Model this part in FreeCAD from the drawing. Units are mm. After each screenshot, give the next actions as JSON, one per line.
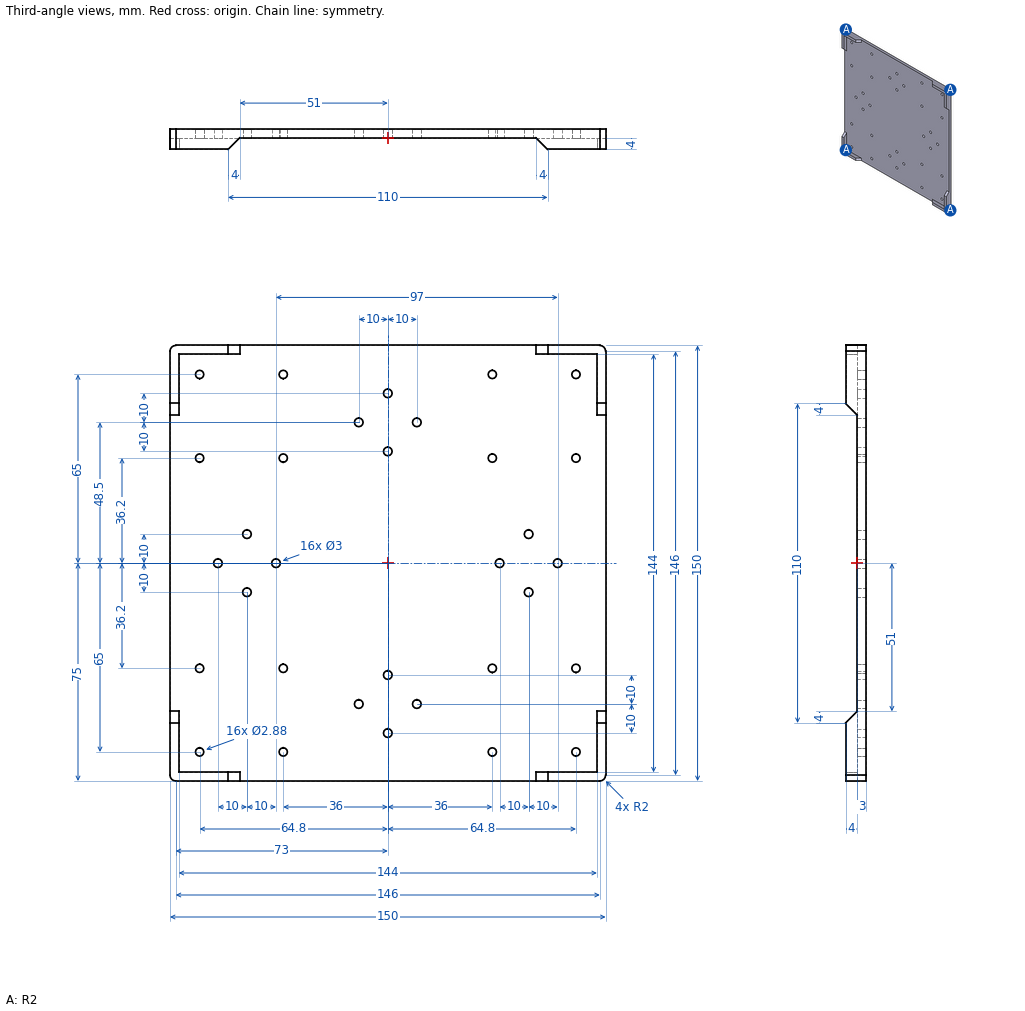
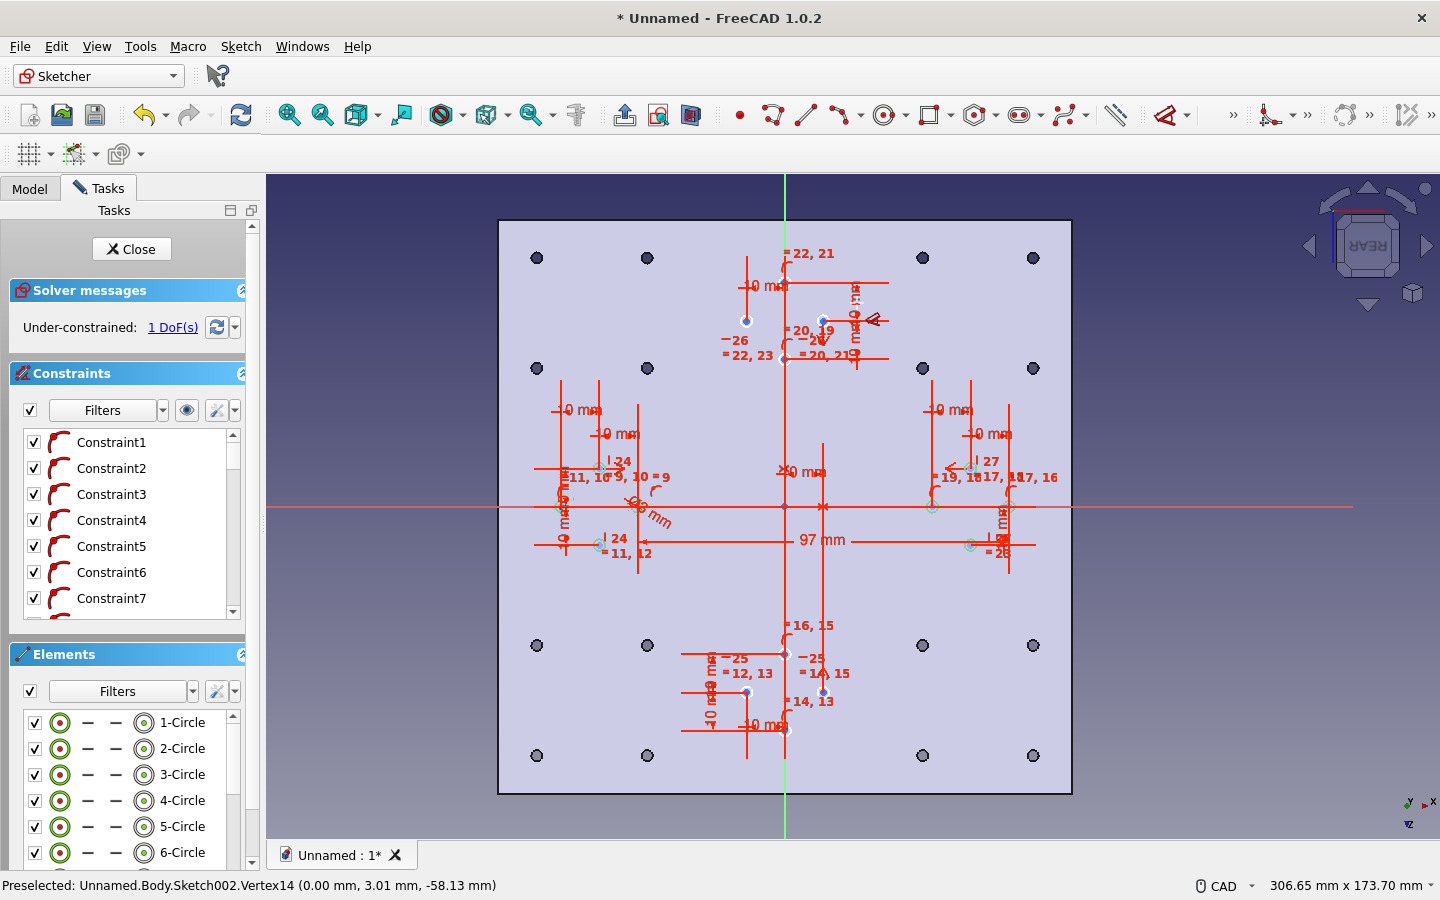
{"action": "left_click", "coordinate": [747, 693]}
{"action": "left_click", "coordinate": [713, 600]}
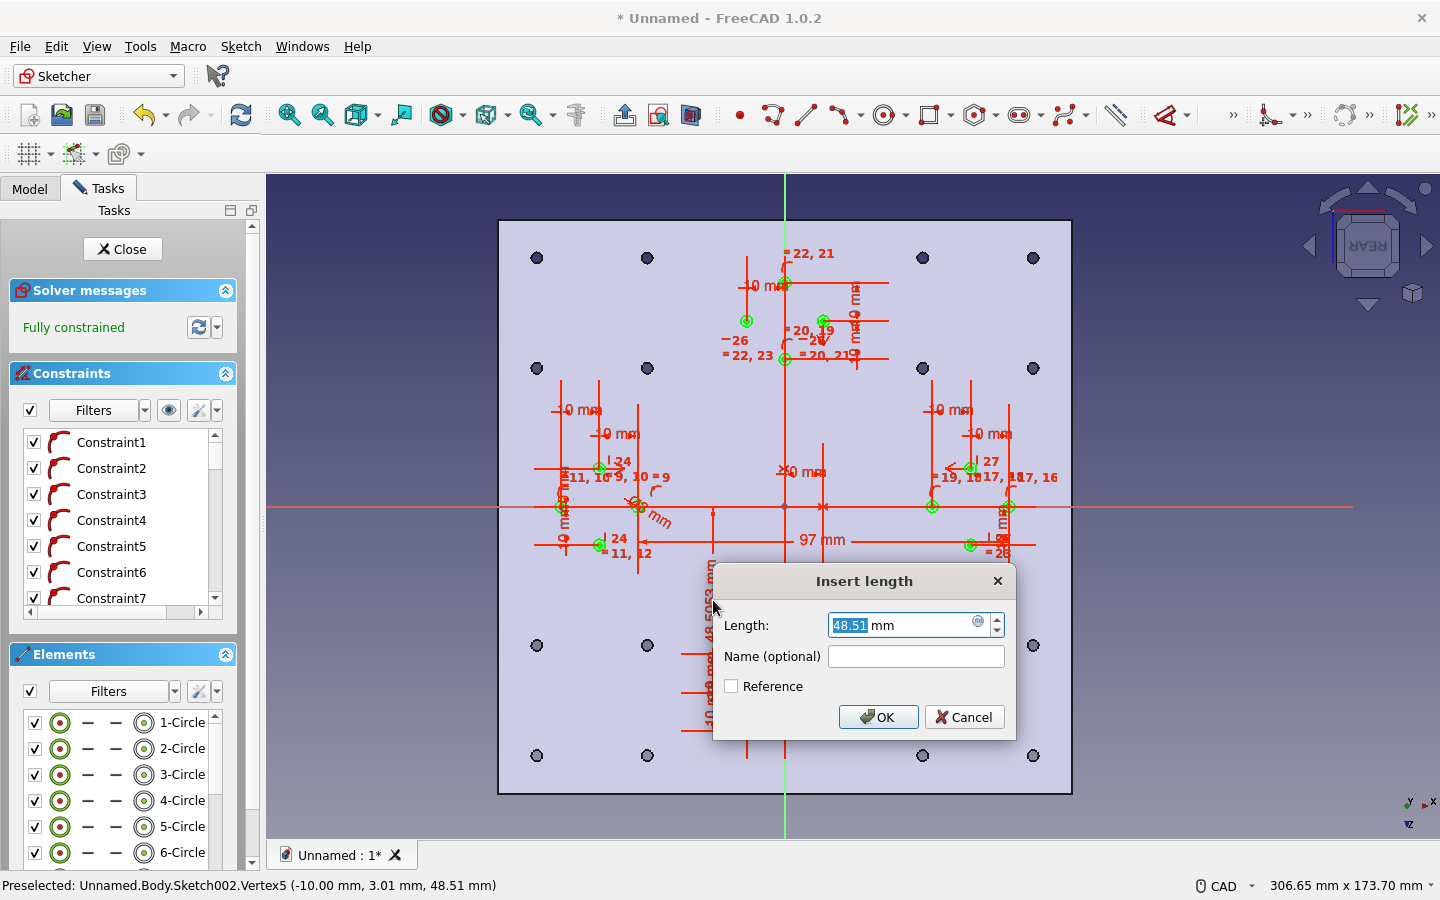
{"action": "type", "text": "48.5"}
{"action": "key", "text": "Return"}
{"action": "key", "text": "Escape"}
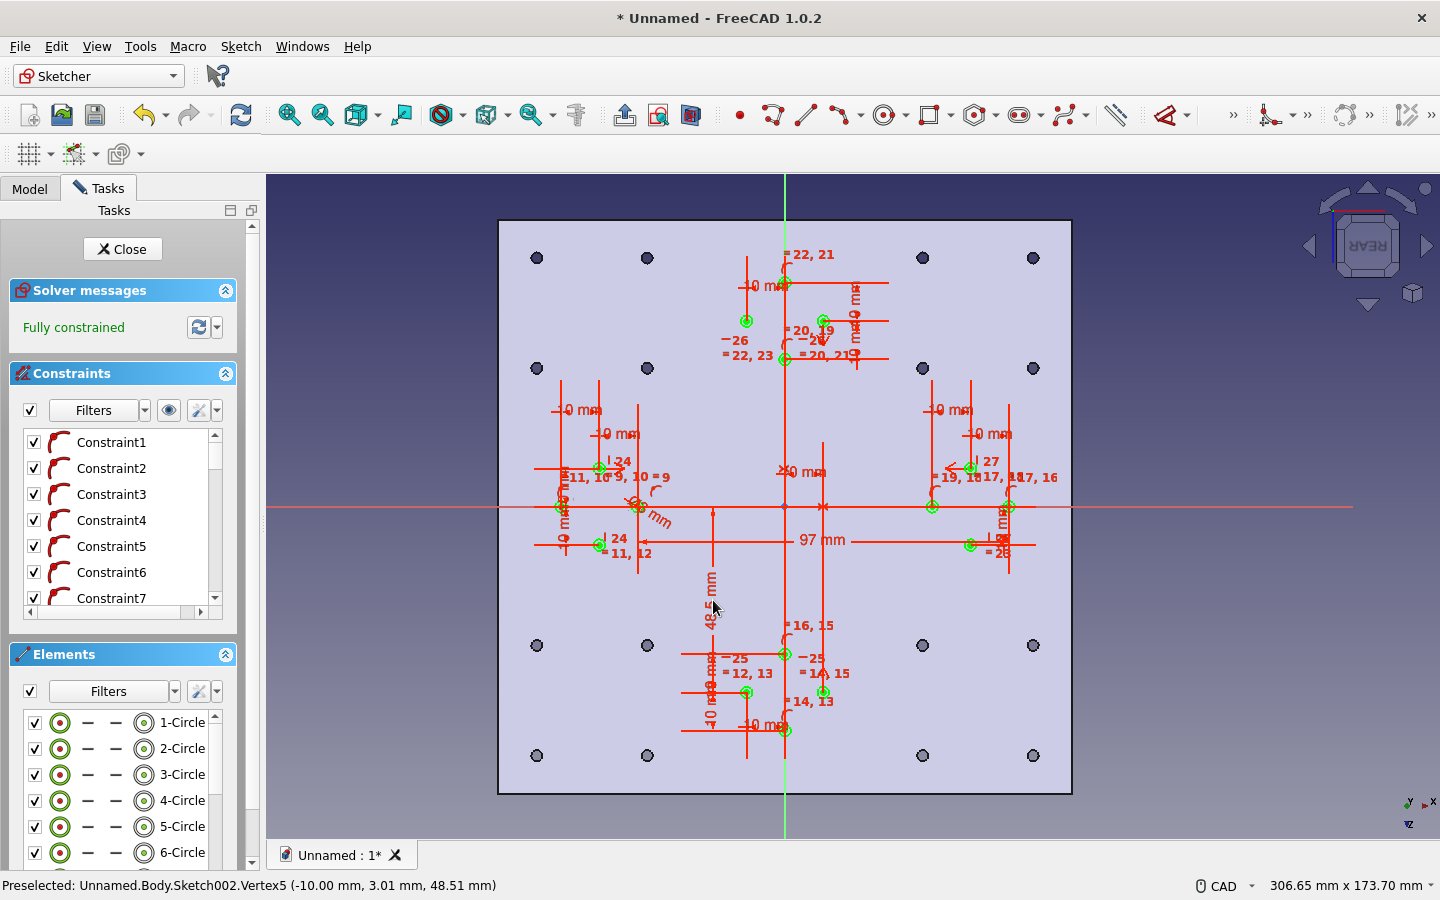
{"action": "left_click", "coordinate": [123, 249]}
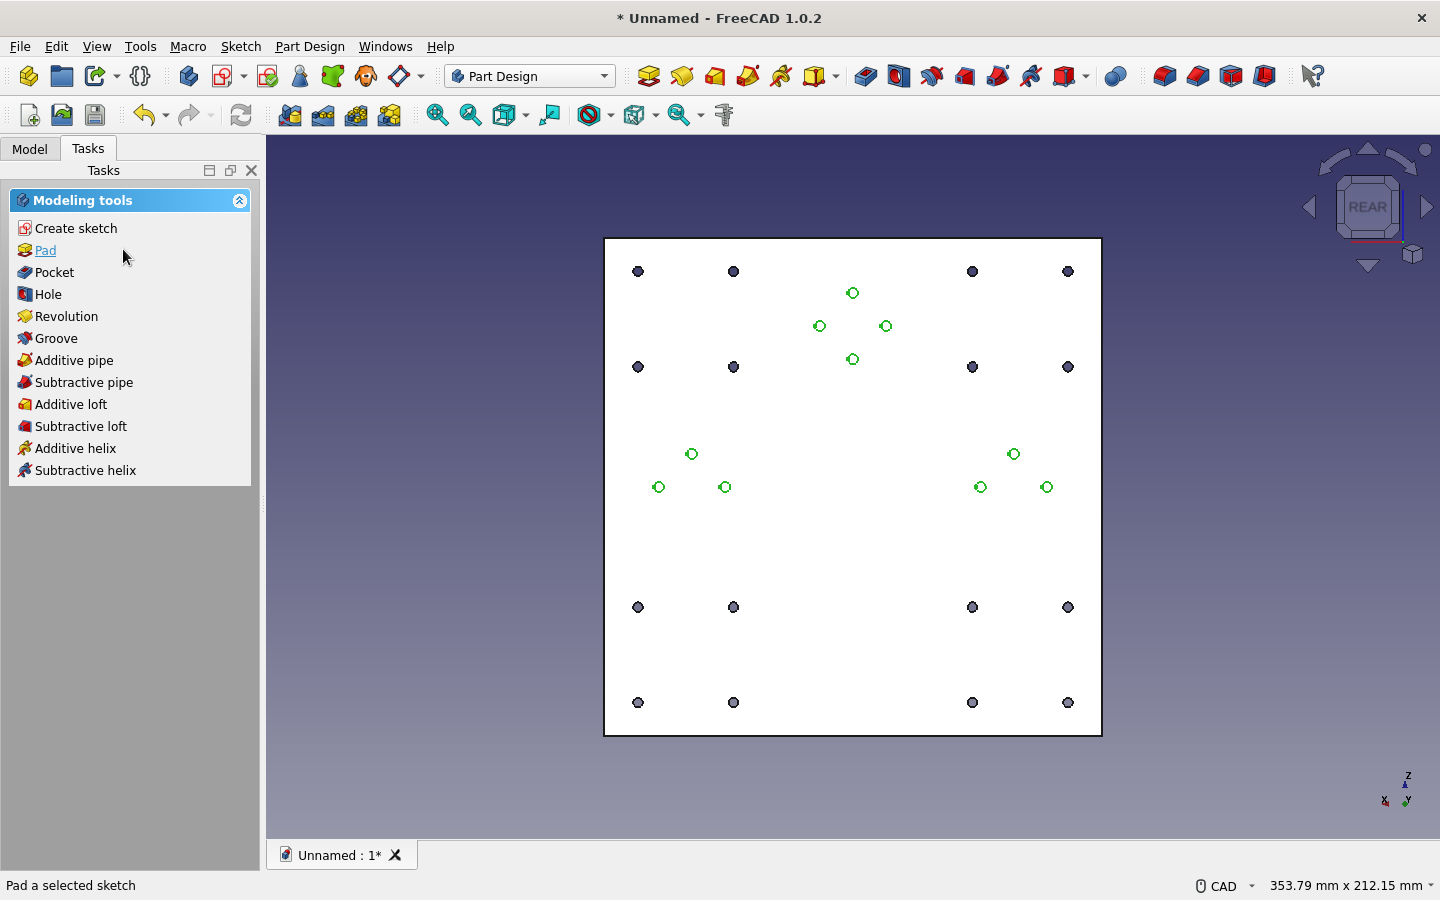
{"action": "left_click", "coordinate": [866, 76]}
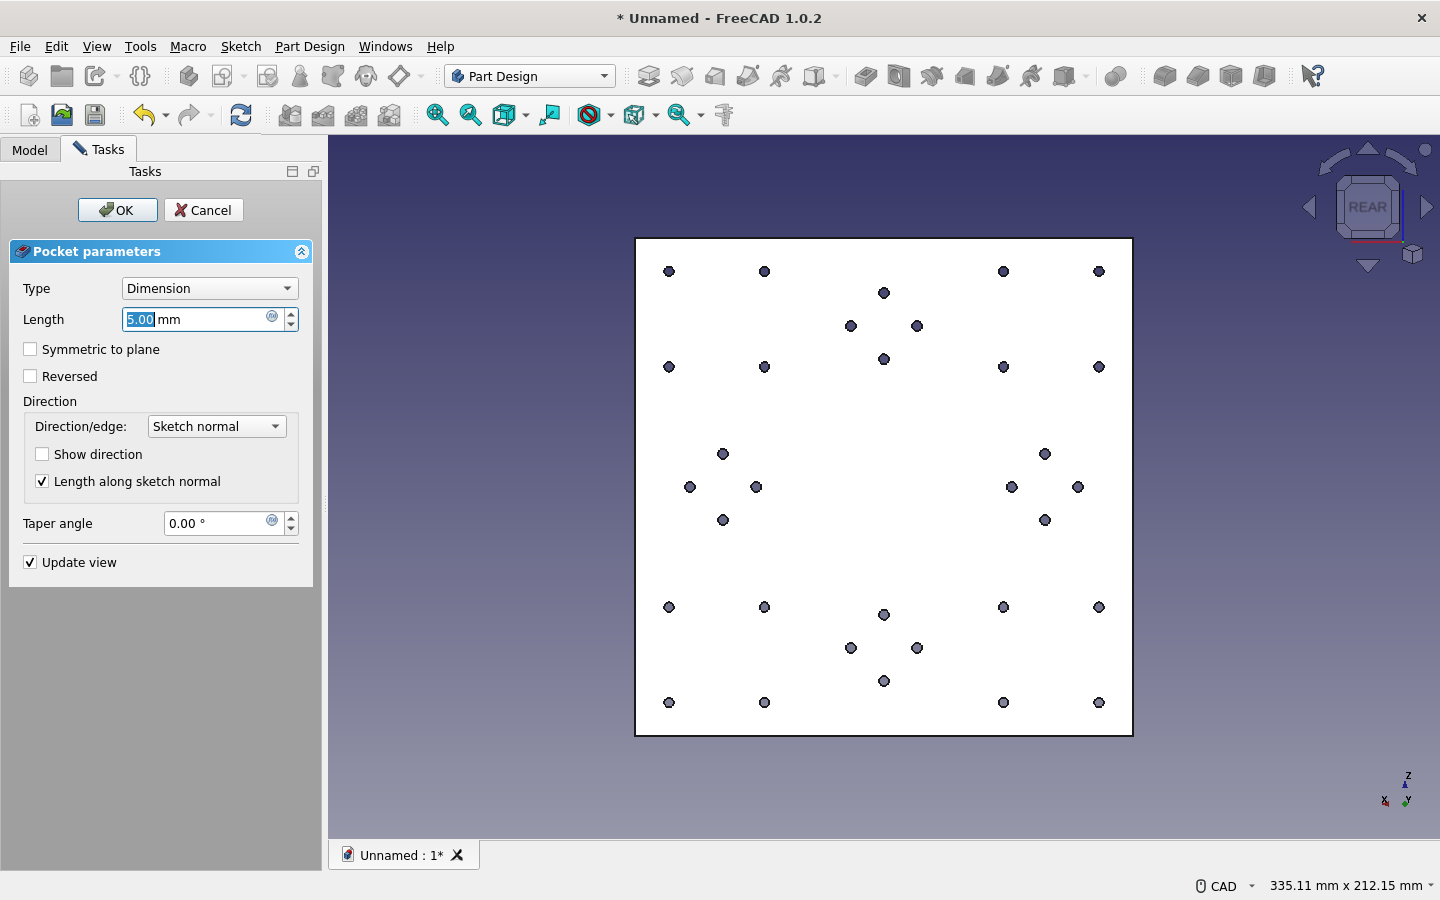
{"action": "left_click", "coordinate": [210, 288]}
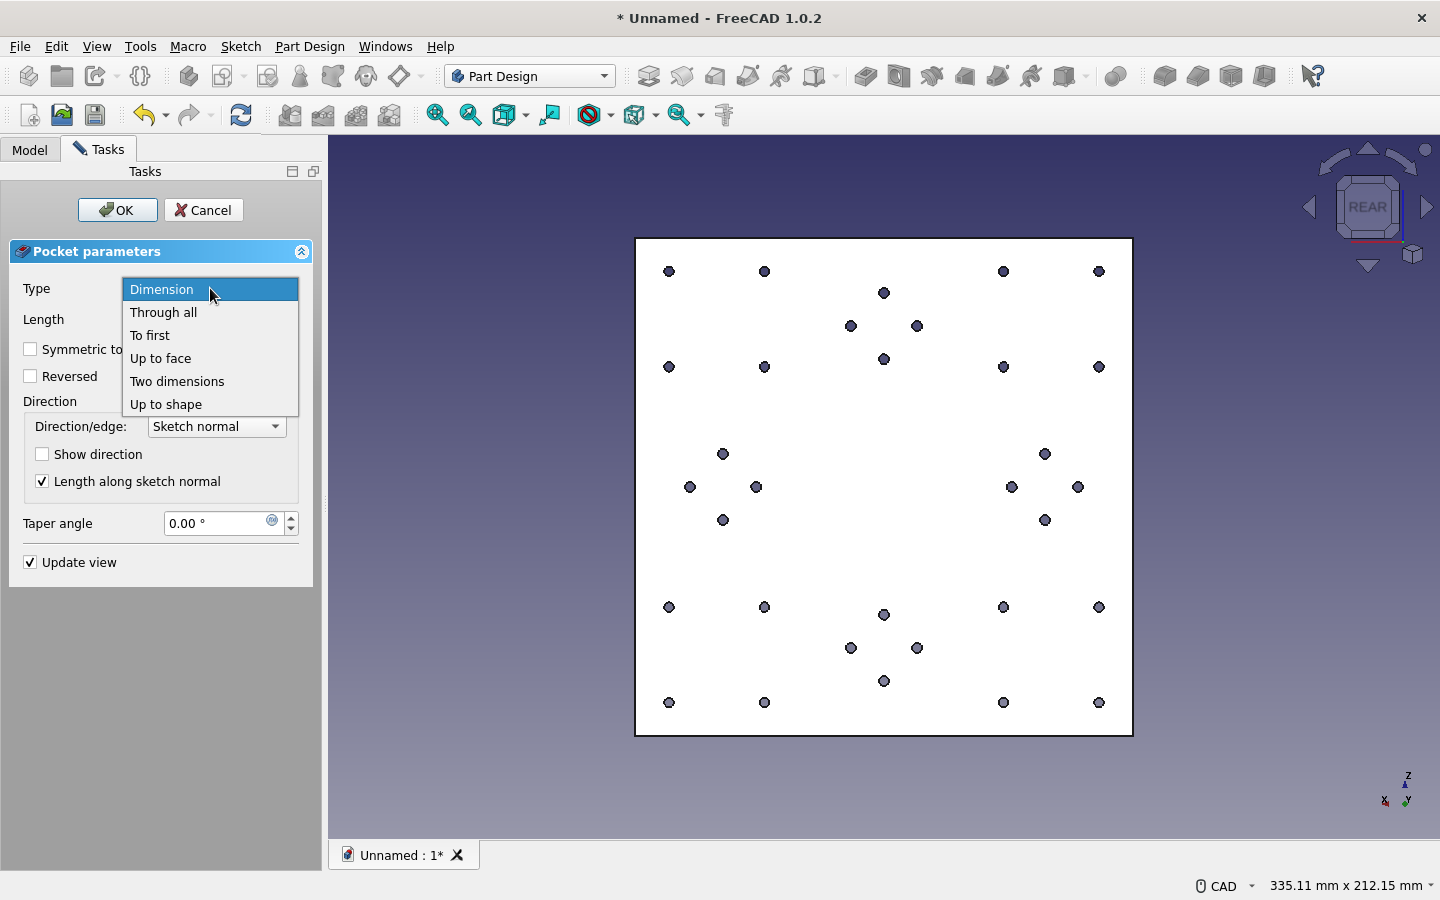
{"action": "left_click", "coordinate": [208, 312]}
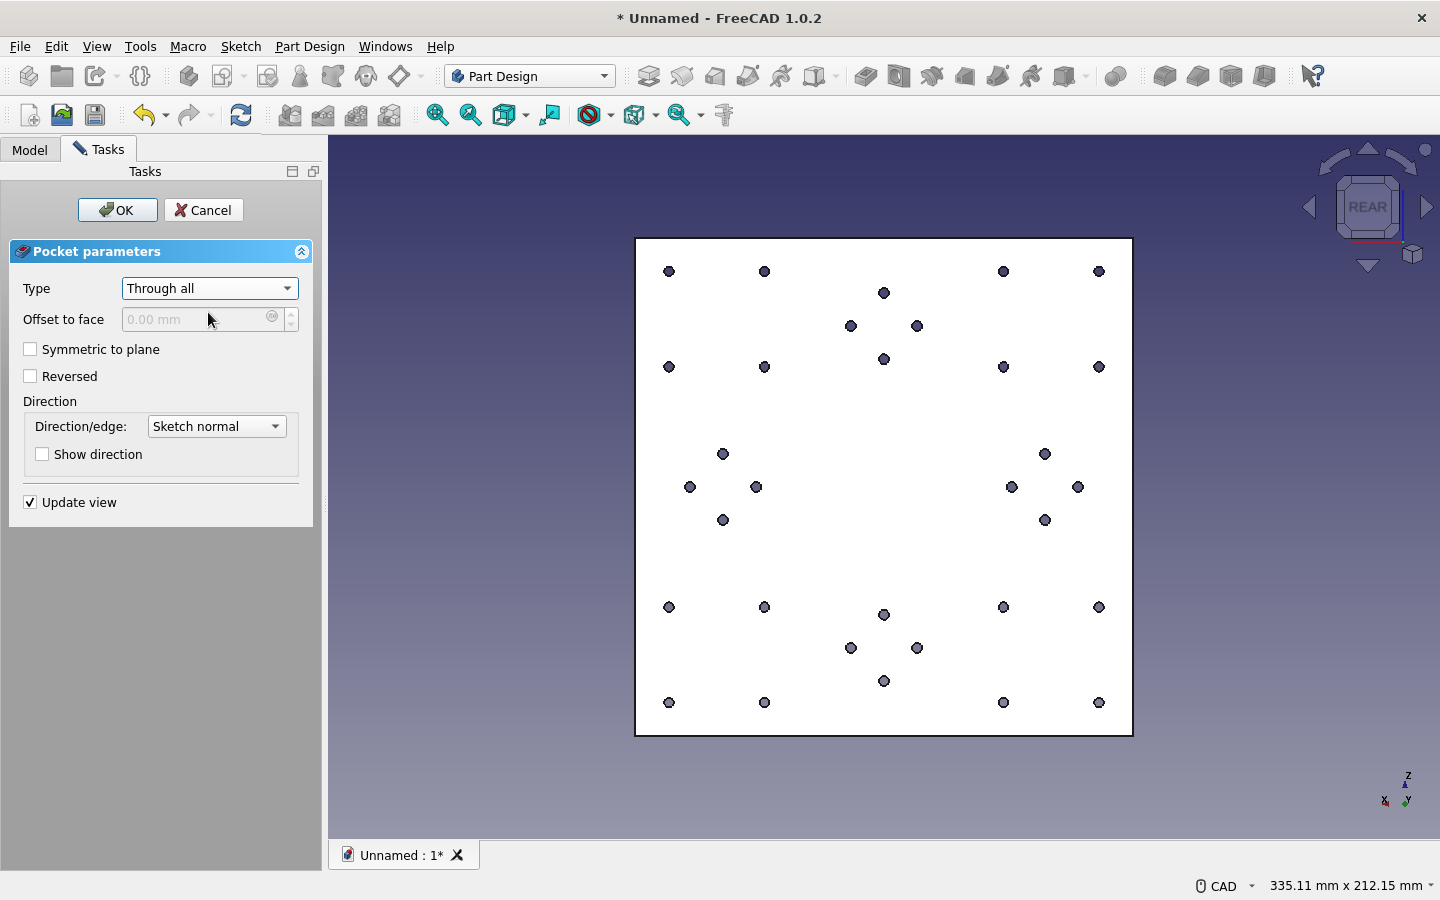
{"action": "left_click", "coordinate": [118, 210]}